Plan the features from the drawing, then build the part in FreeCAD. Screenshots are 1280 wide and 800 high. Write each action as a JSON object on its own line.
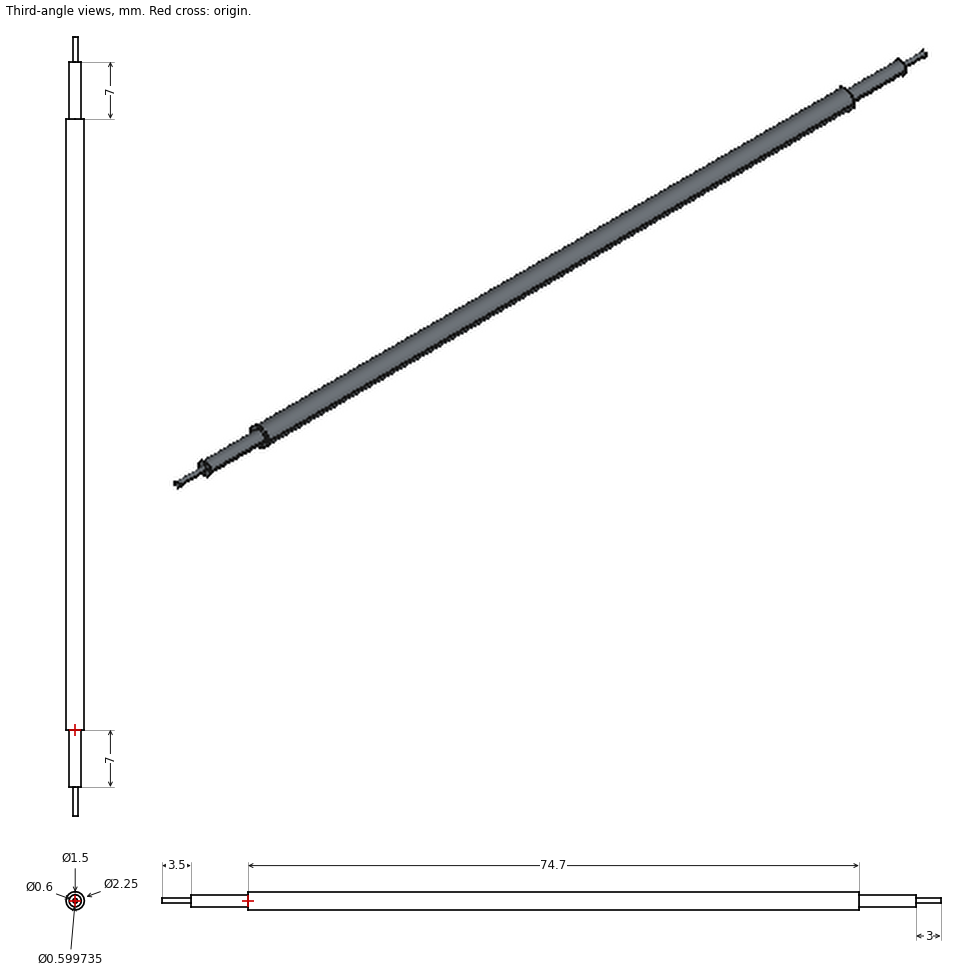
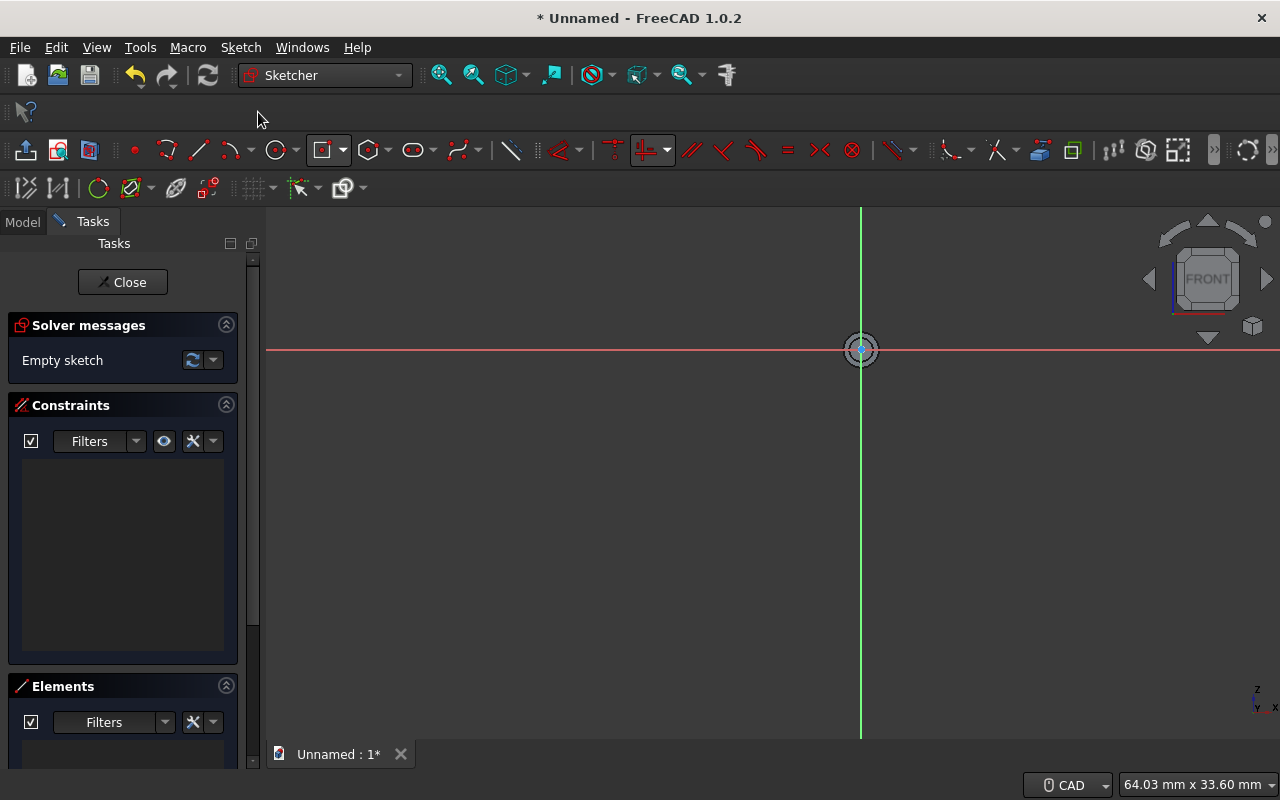
{"action": "scroll", "coordinate": [869, 343], "scroll_direction": "up", "scroll_amount": 15}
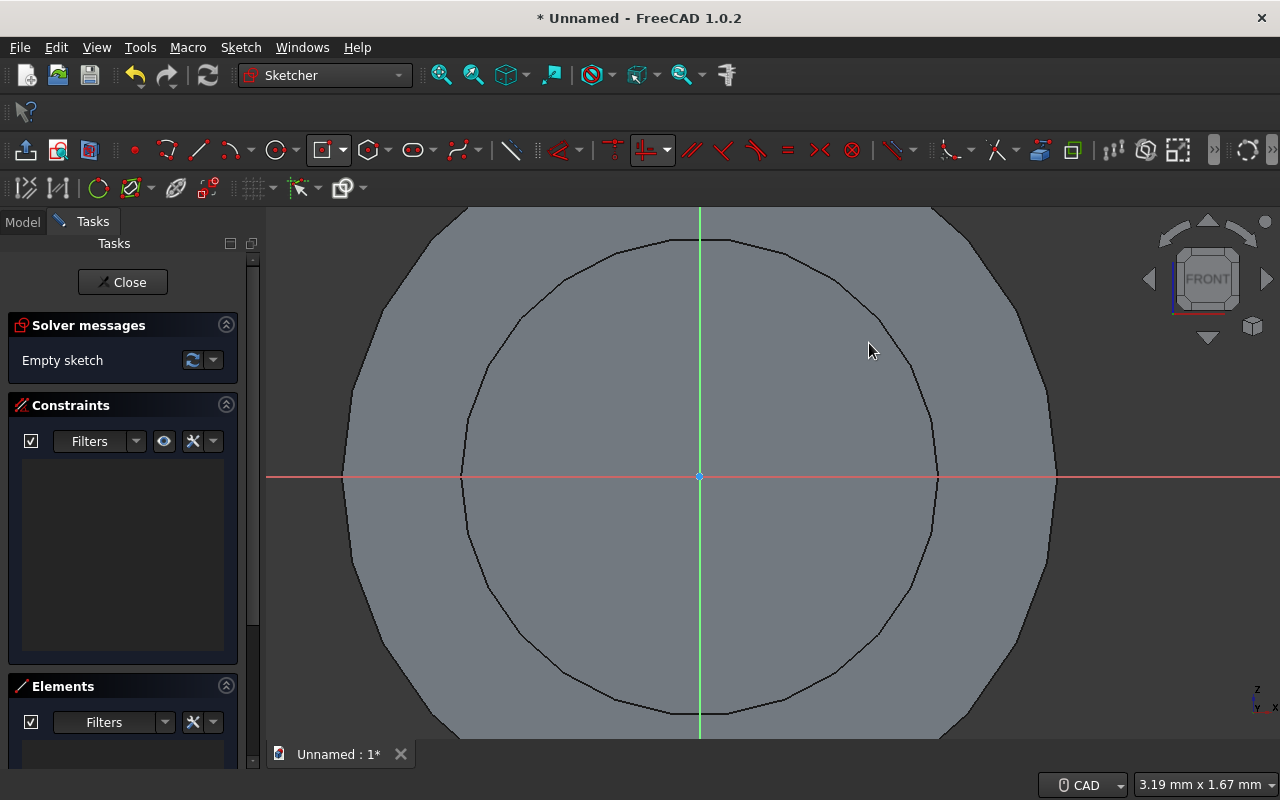
{"action": "scroll", "coordinate": [694, 481], "scroll_direction": "up", "scroll_amount": 3}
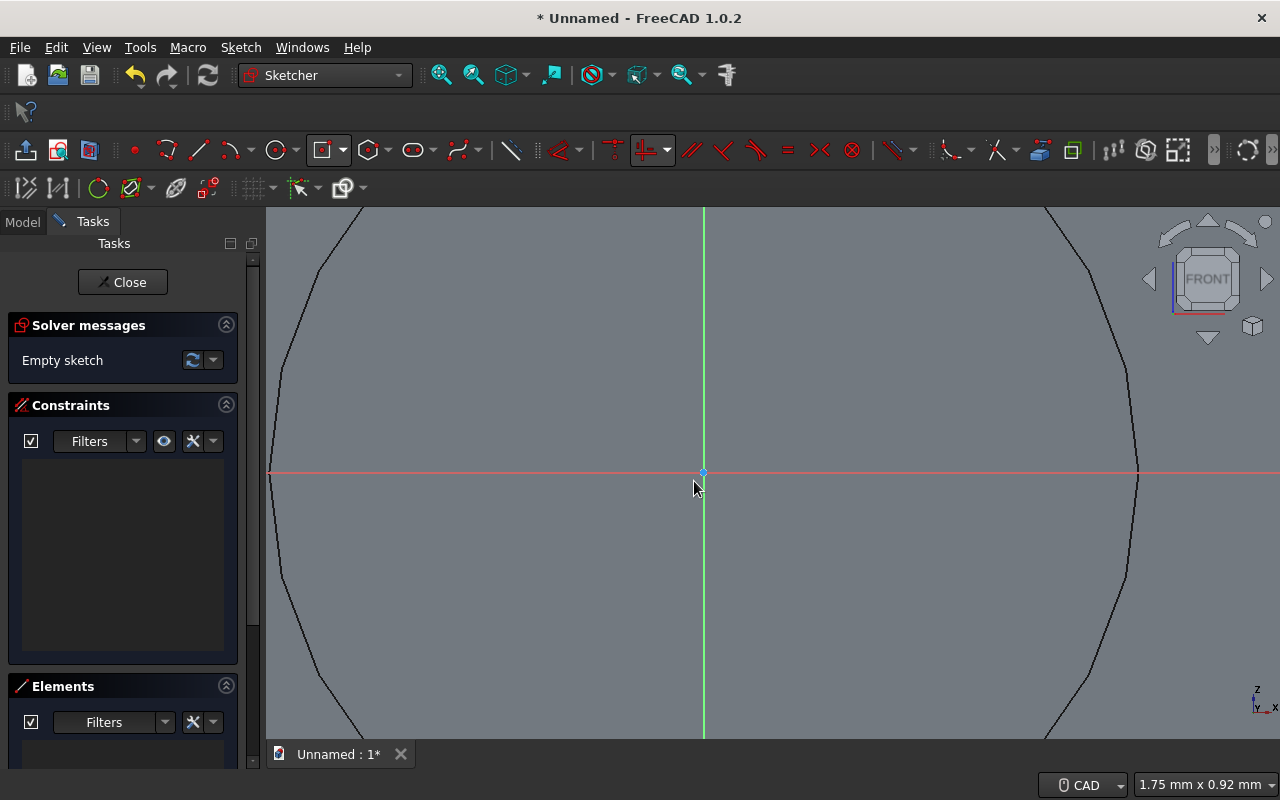
{"action": "left_click", "coordinate": [276, 150]}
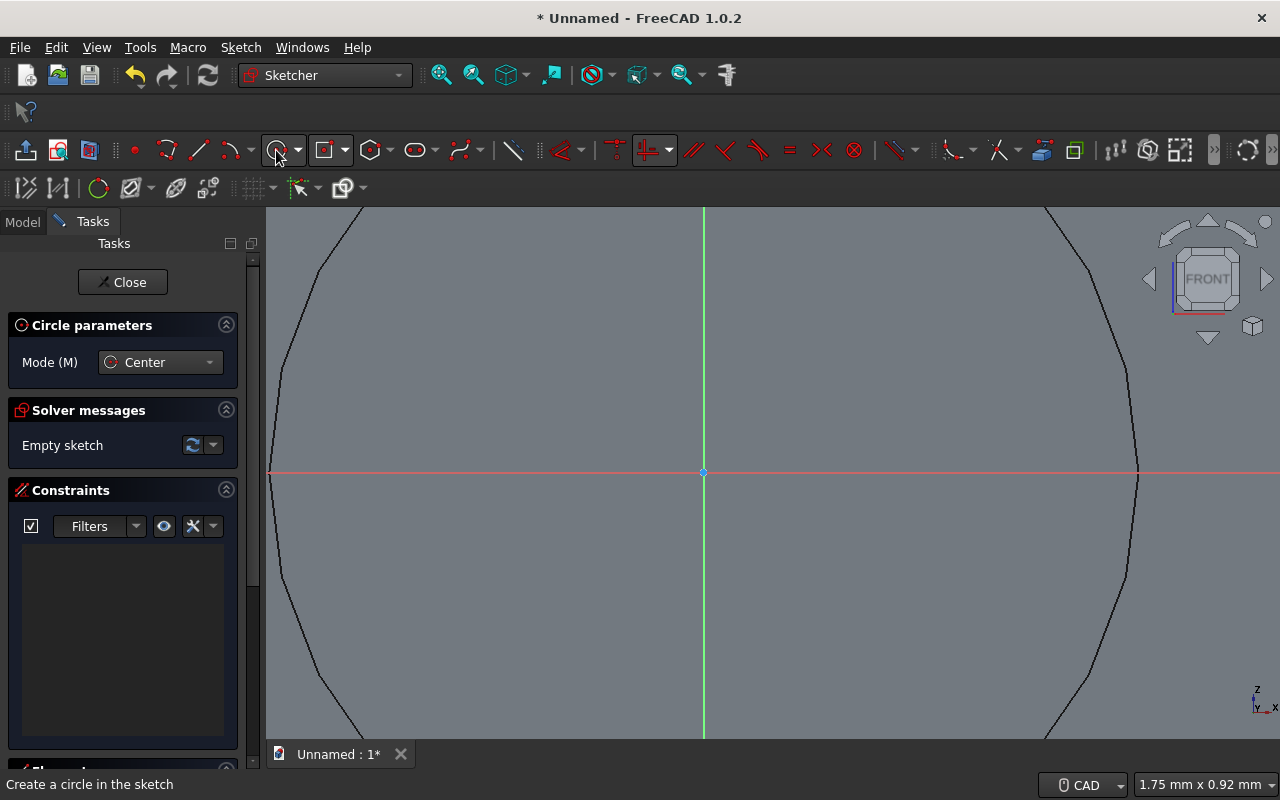
{"action": "left_click", "coordinate": [704, 473]}
{"action": "mouse_move", "coordinate": [827, 350]}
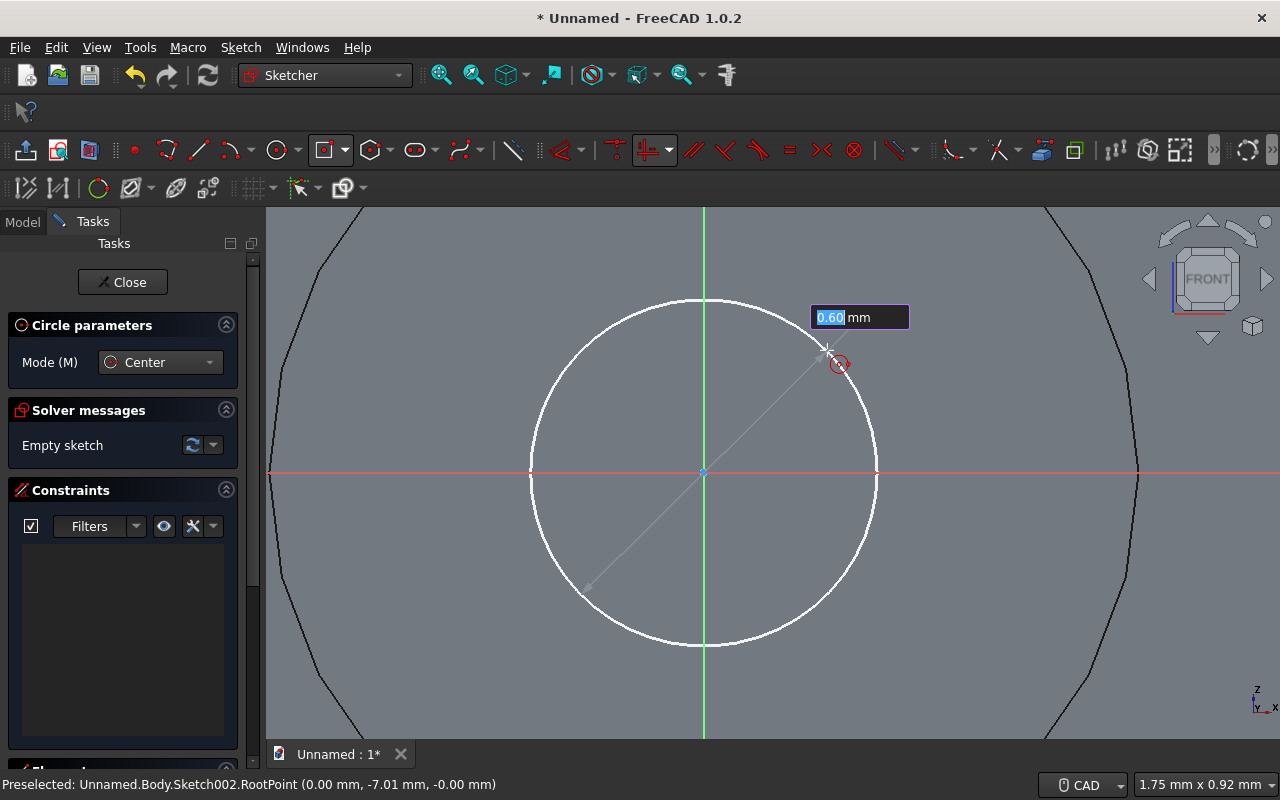
{"action": "type", "text": "0.6"}
{"action": "key", "text": "Return"}
{"action": "key", "text": "Escape"}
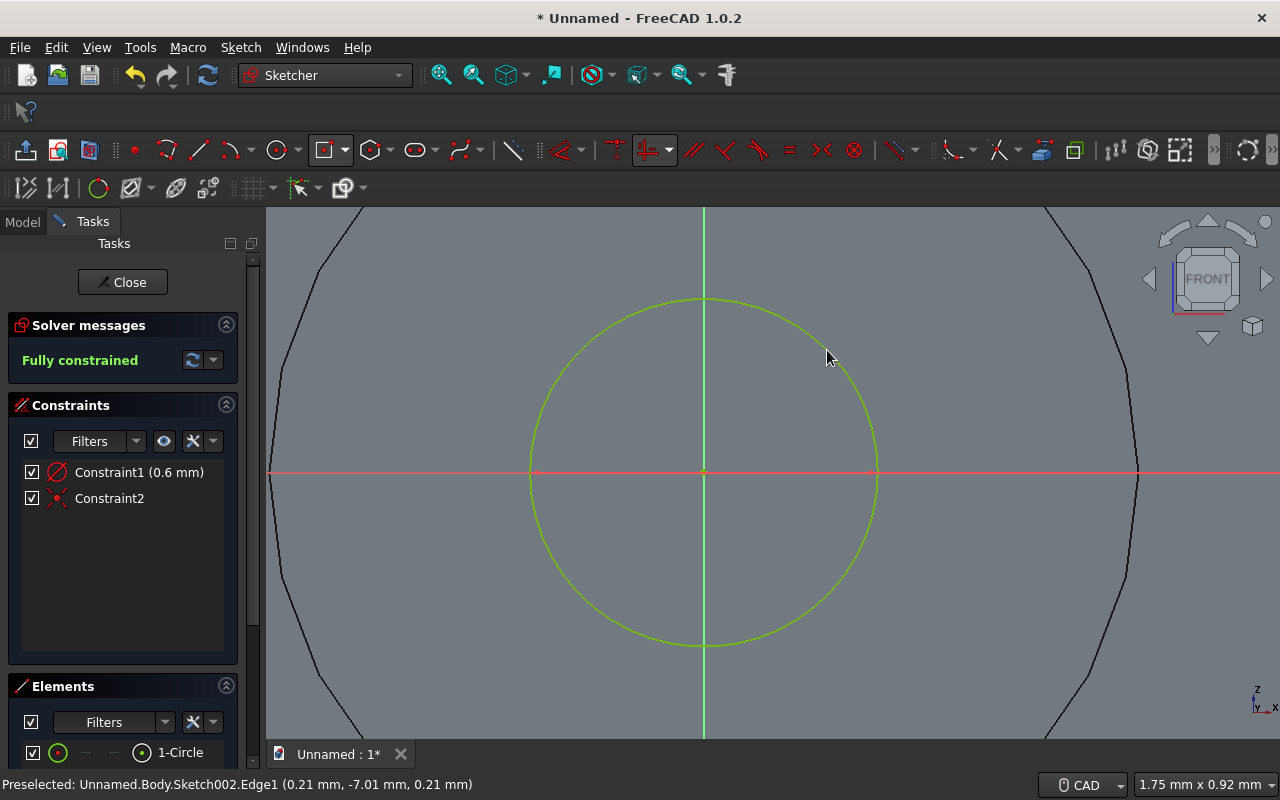
{"action": "left_click", "coordinate": [123, 282]}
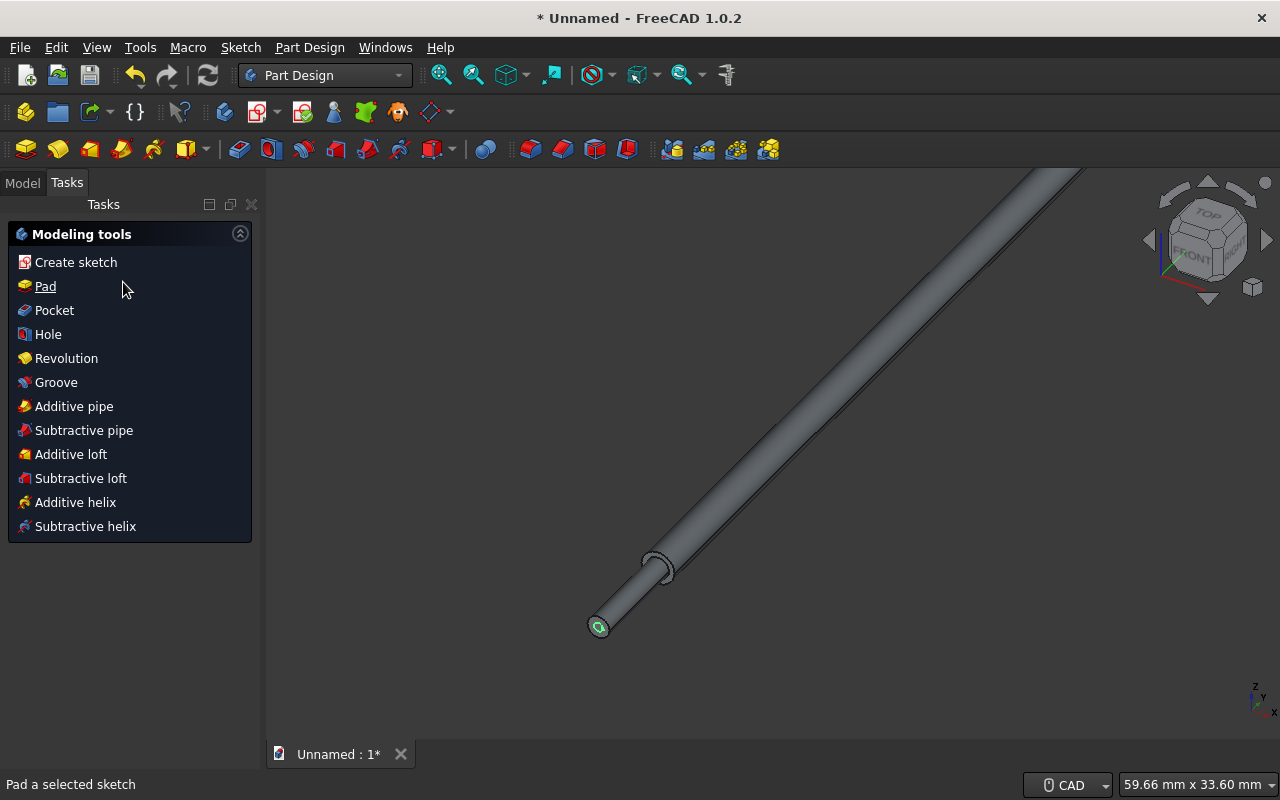
{"action": "left_click", "coordinate": [26, 150]}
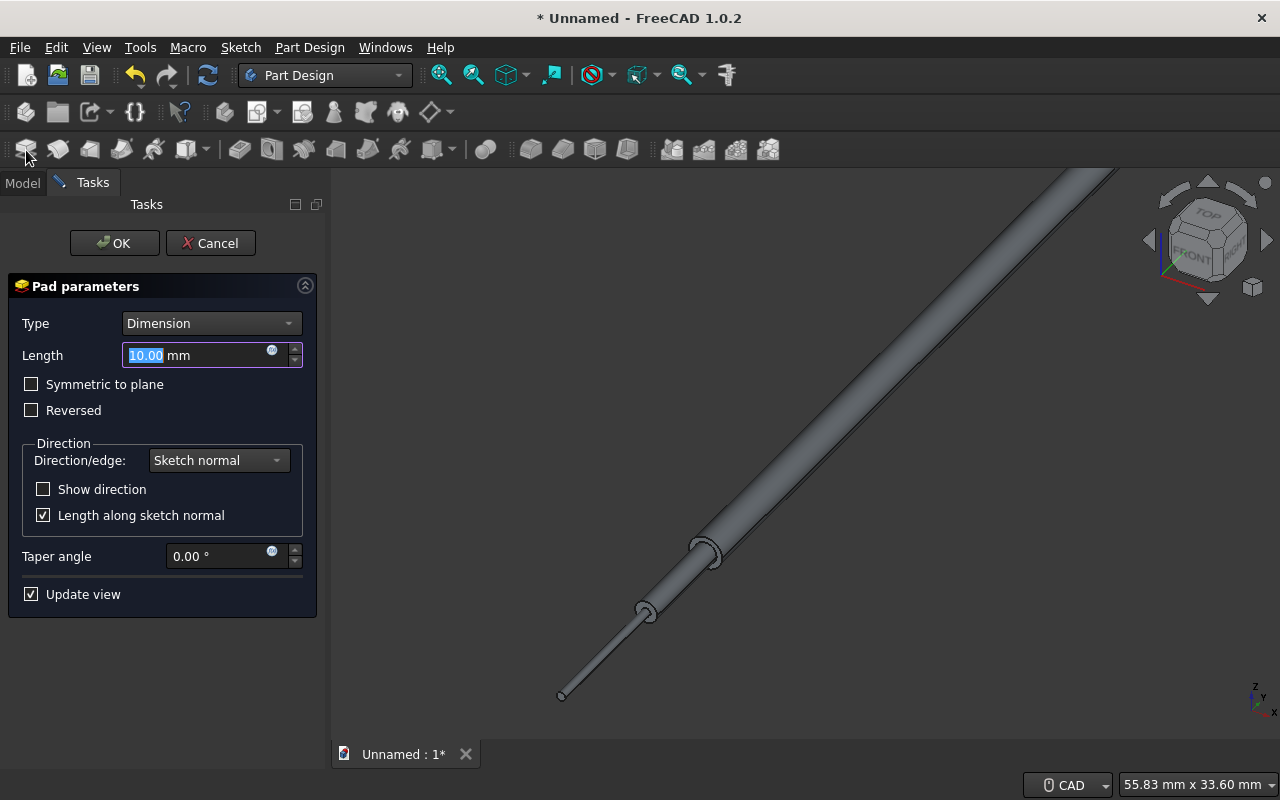
{"action": "type", "text": "3.5"}
{"action": "key", "text": "Tab"}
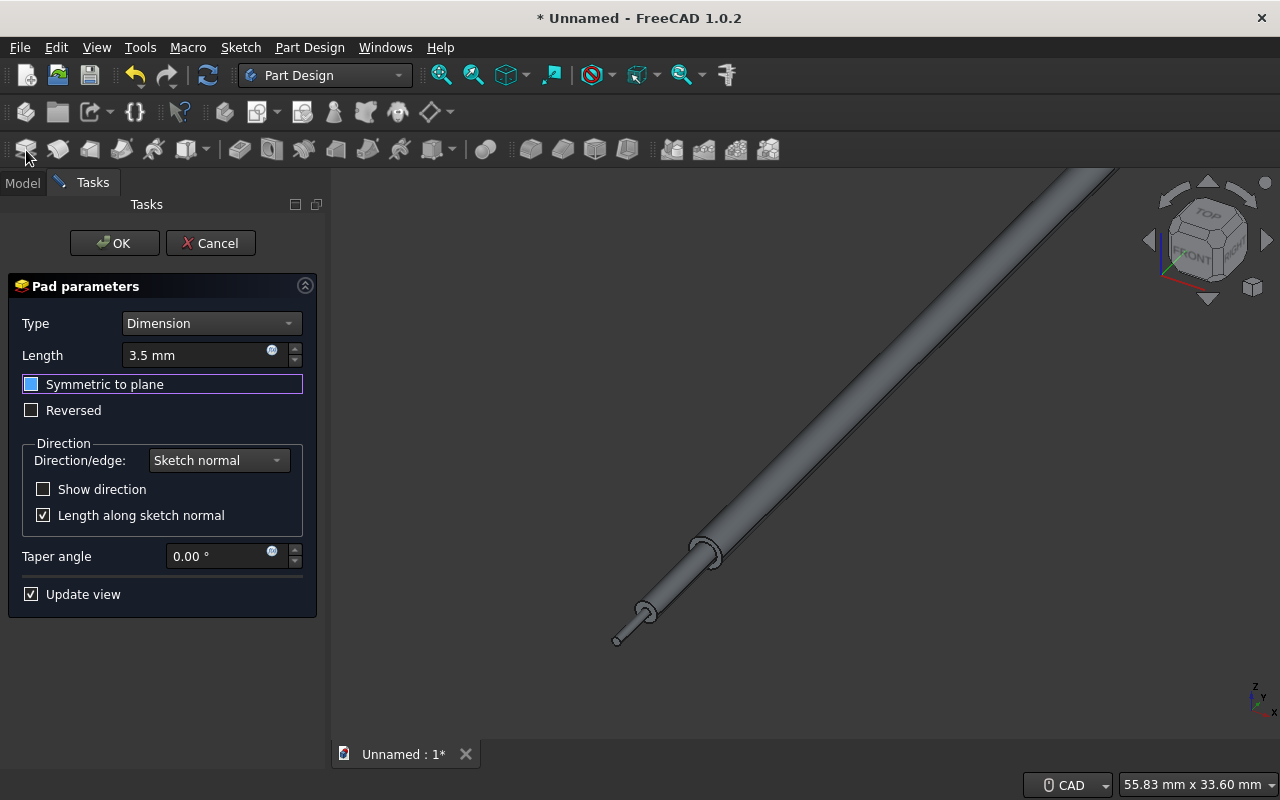
{"action": "left_click", "coordinate": [115, 243]}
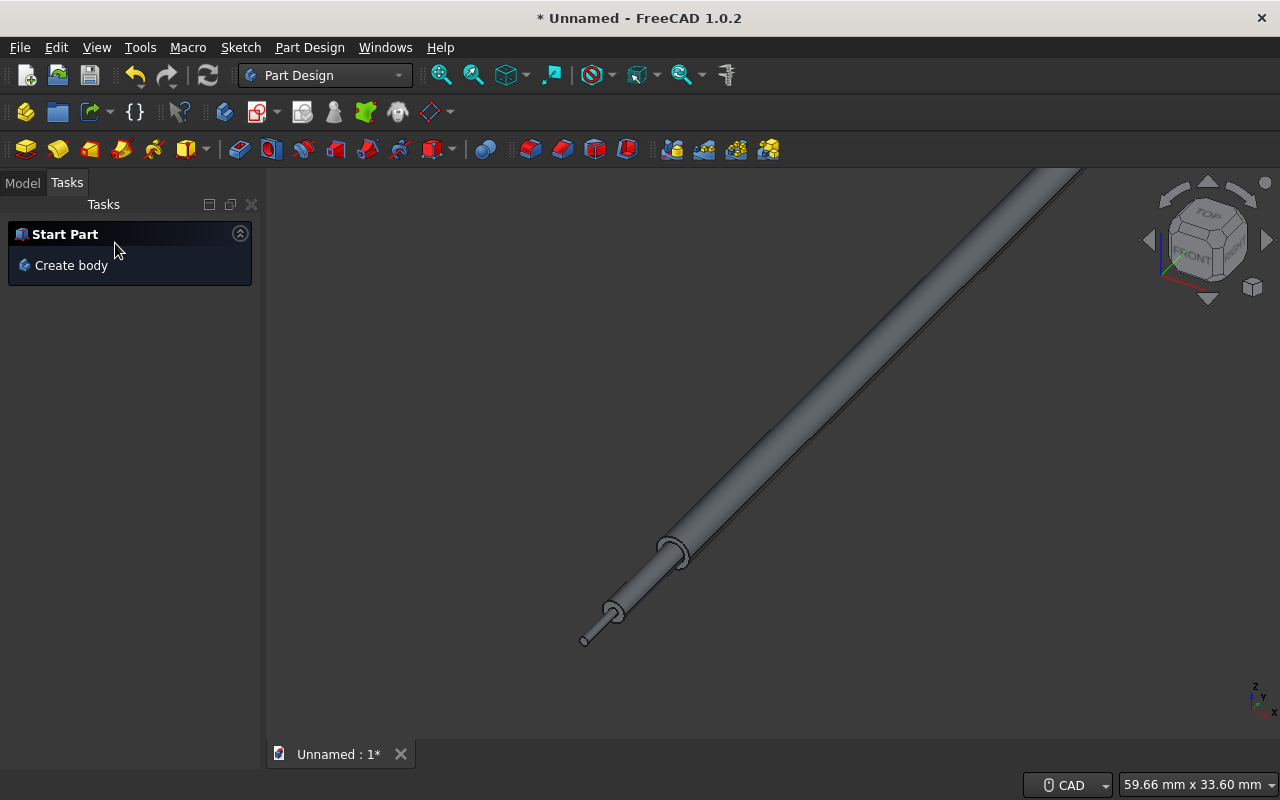
{"action": "left_click", "coordinate": [442, 76]}